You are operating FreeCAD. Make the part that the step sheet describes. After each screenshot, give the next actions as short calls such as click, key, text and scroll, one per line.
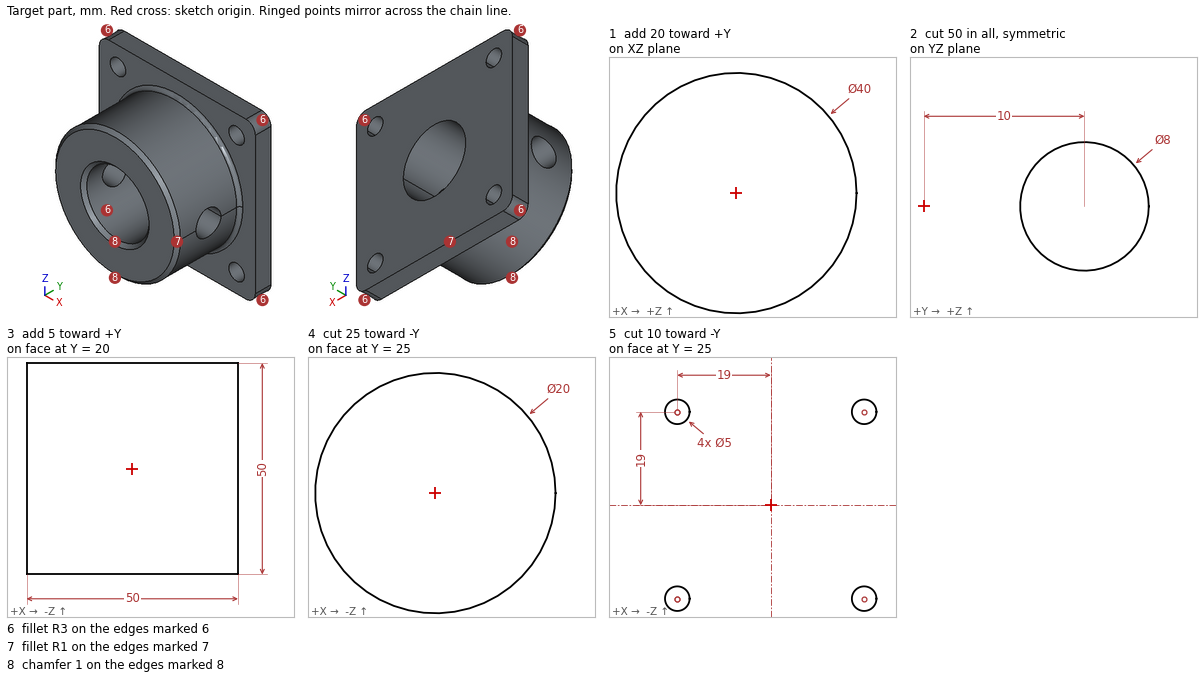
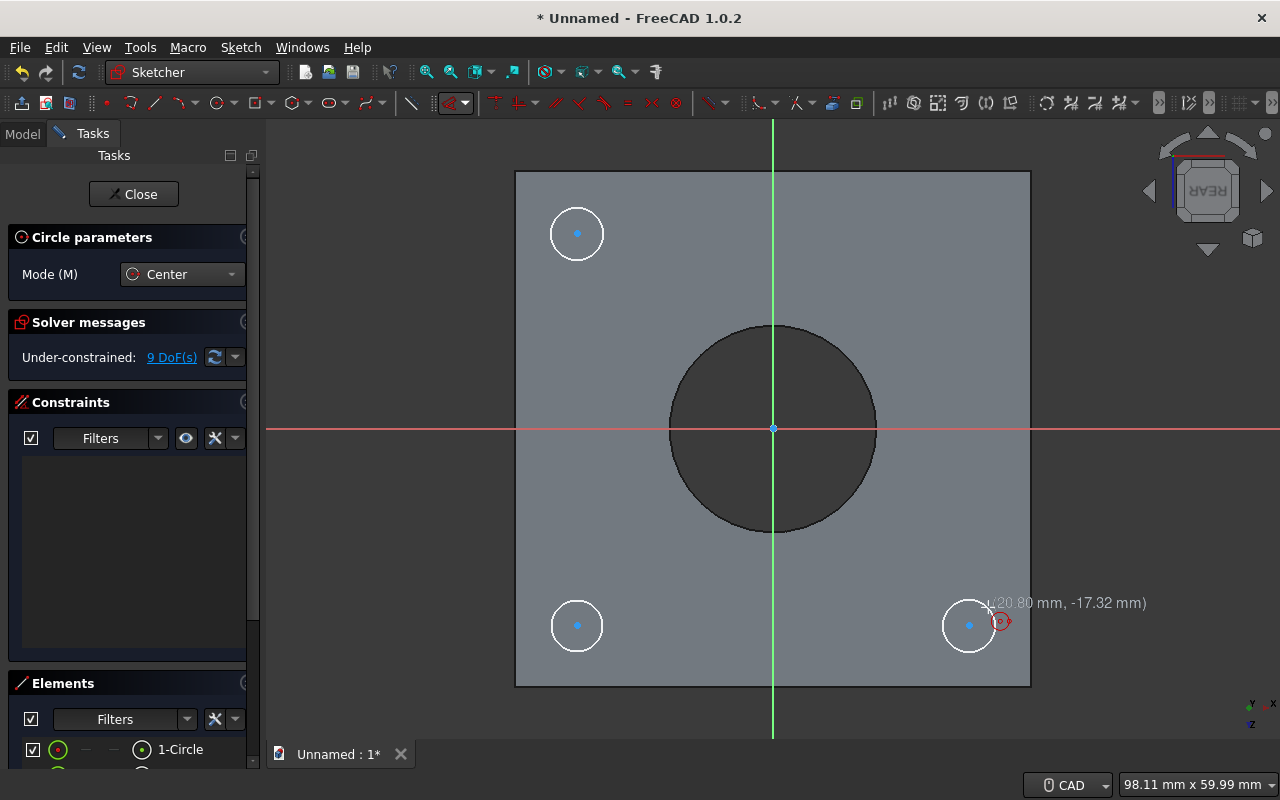
click(969, 233)
click(988, 214)
key(Escape)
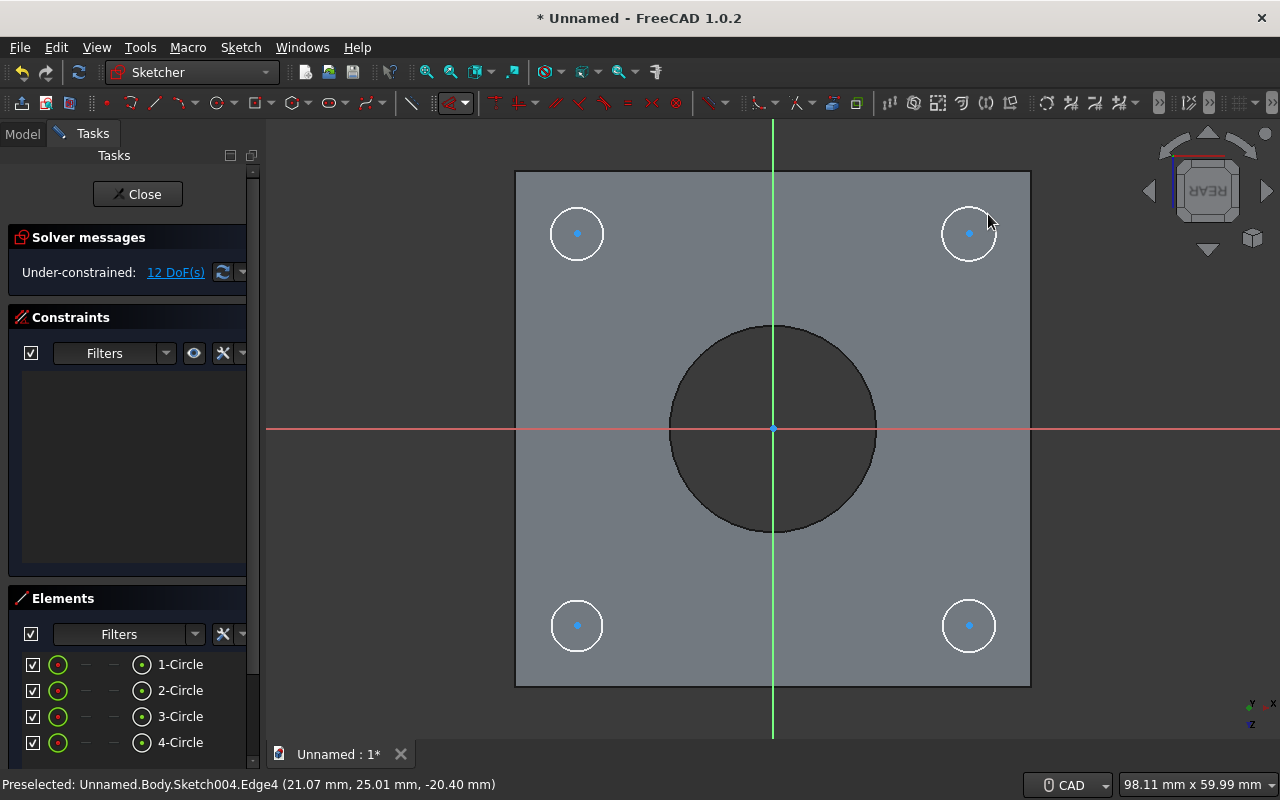
click(595, 215)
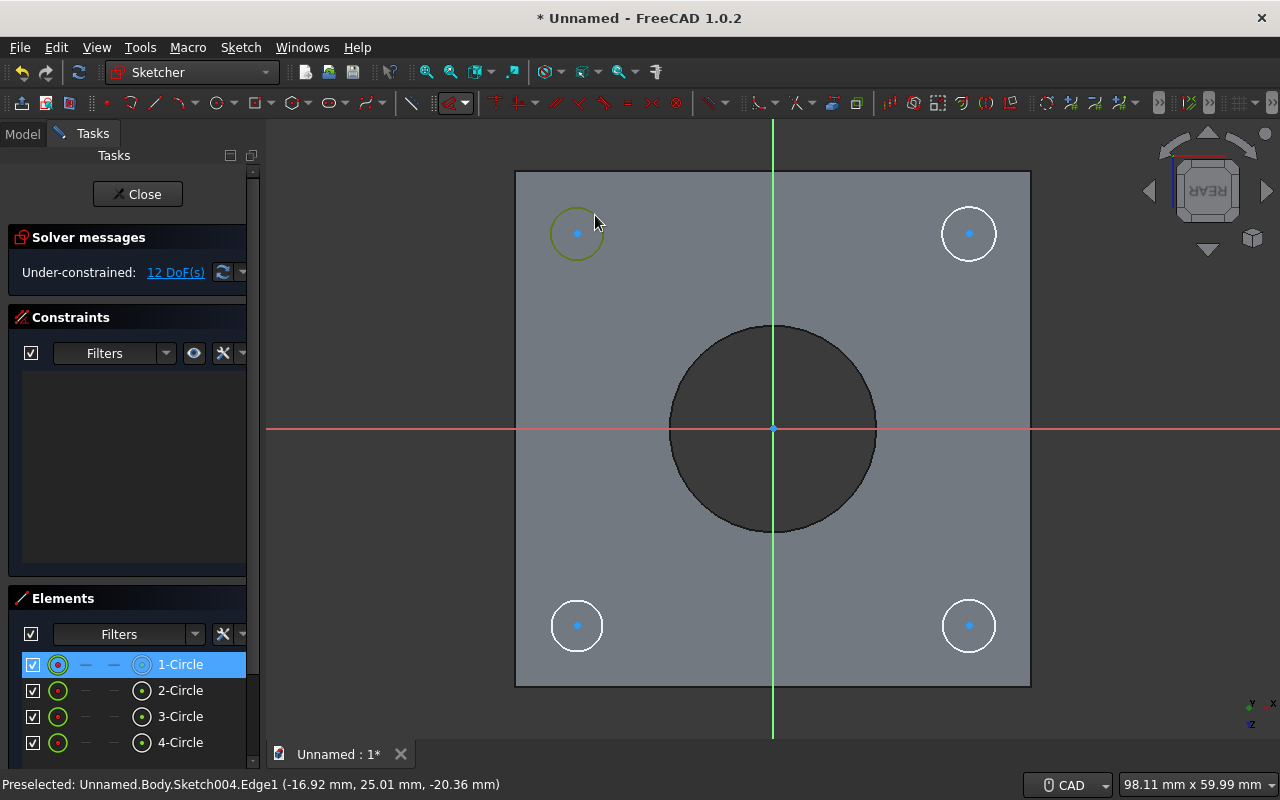
click(595, 608)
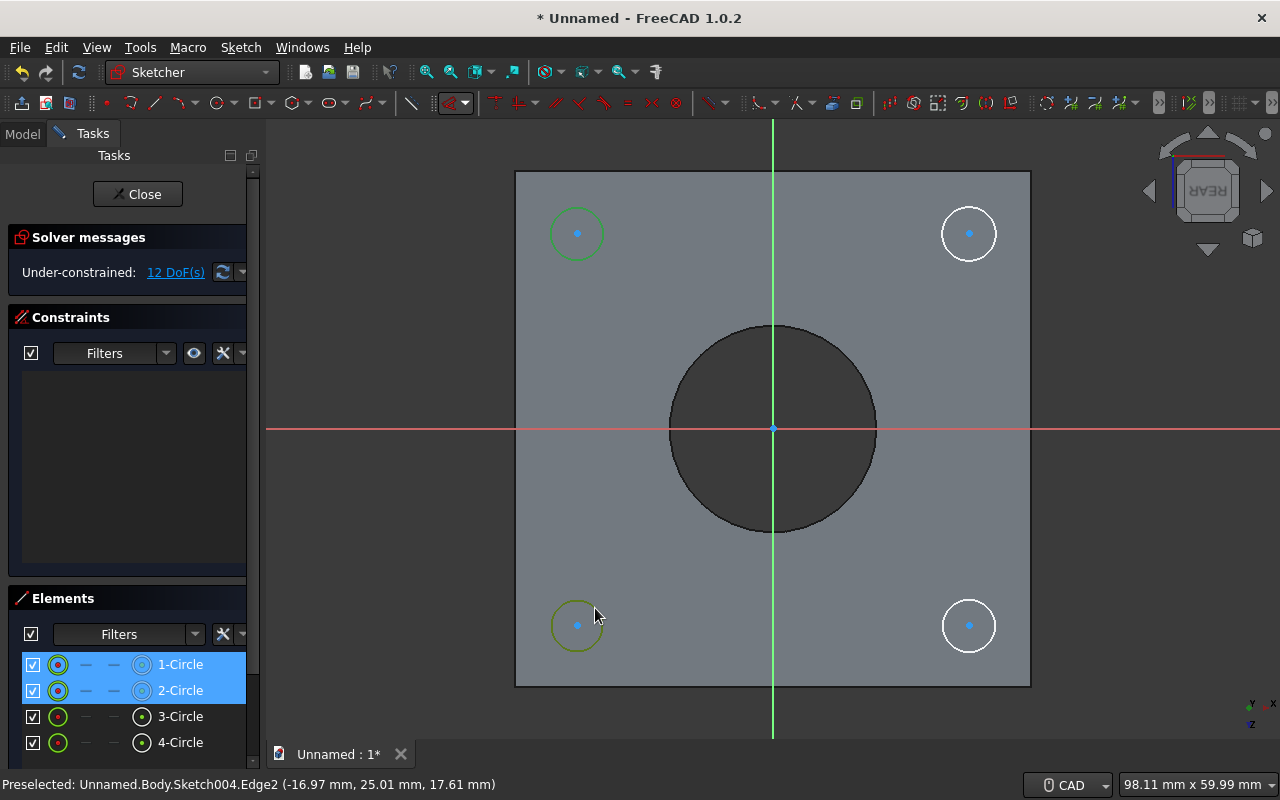
click(987, 607)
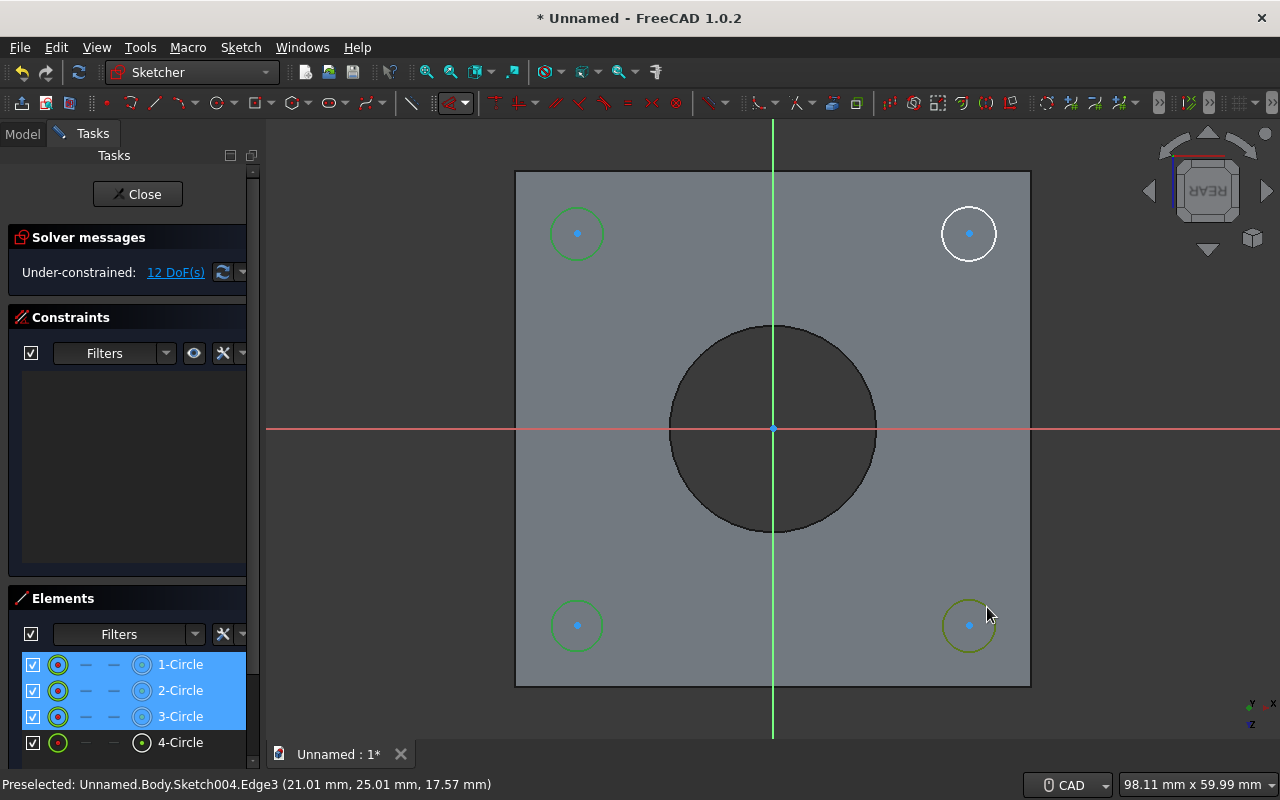
click(988, 215)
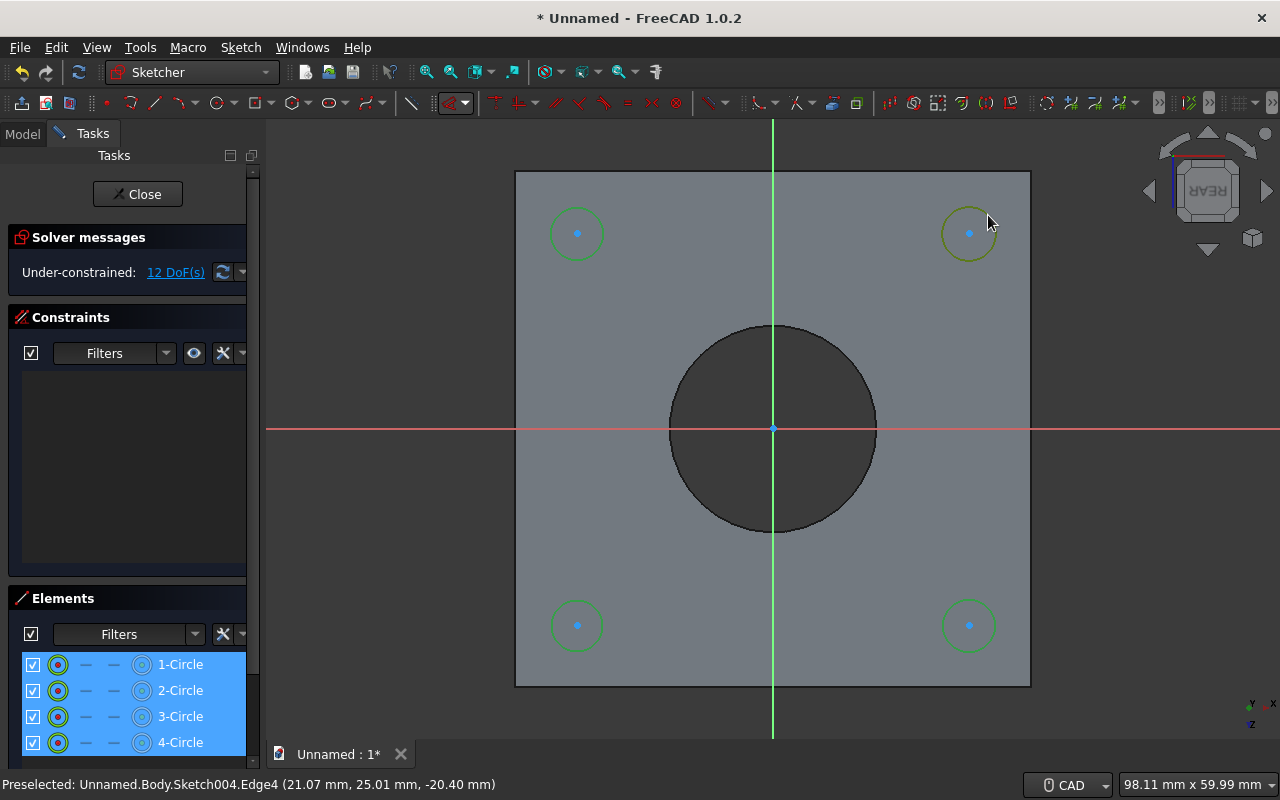
click(628, 104)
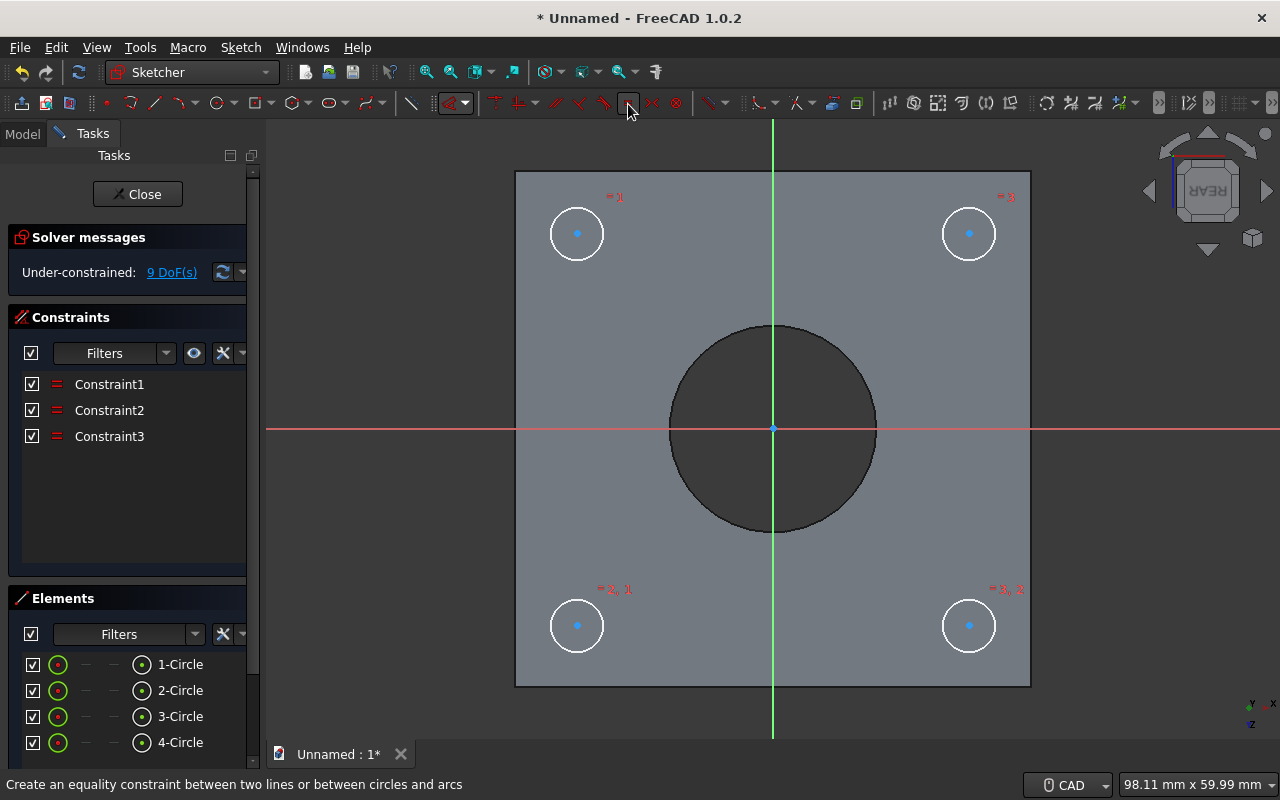
click(577, 234)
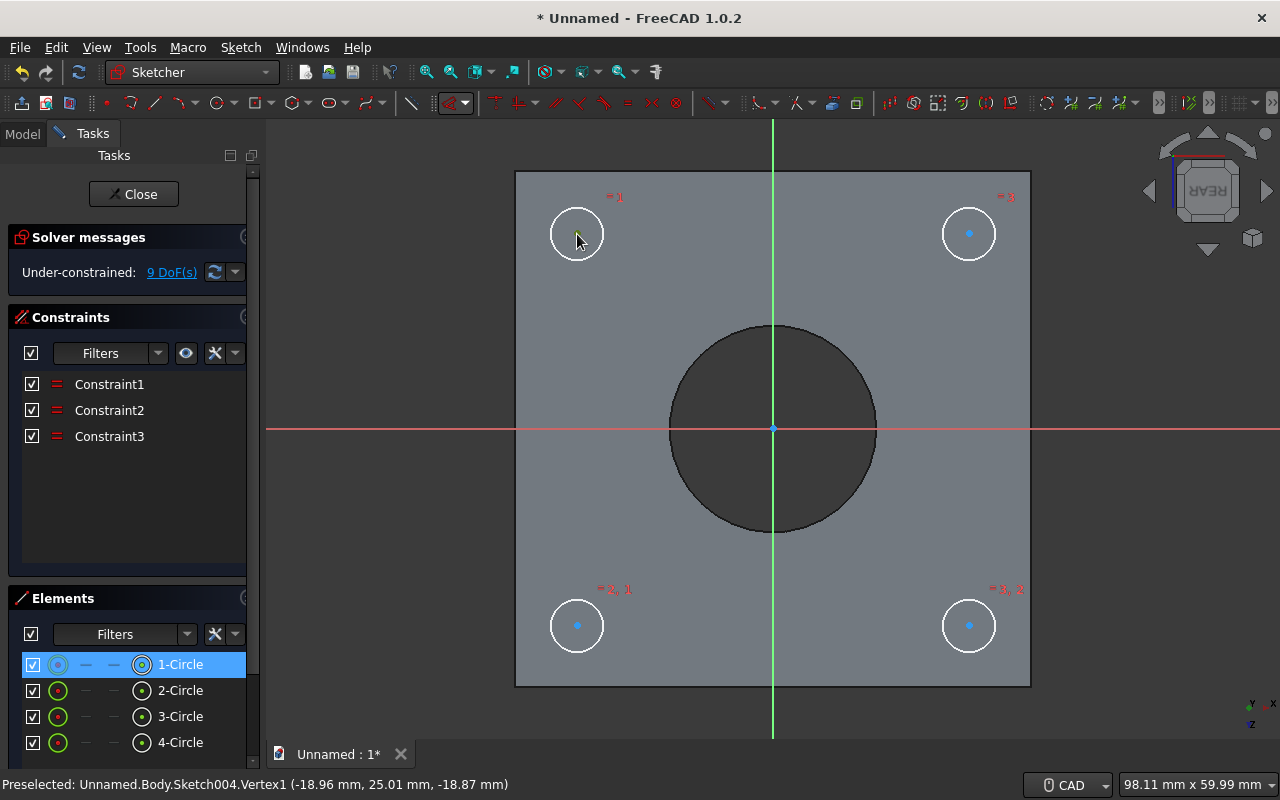
click(577, 626)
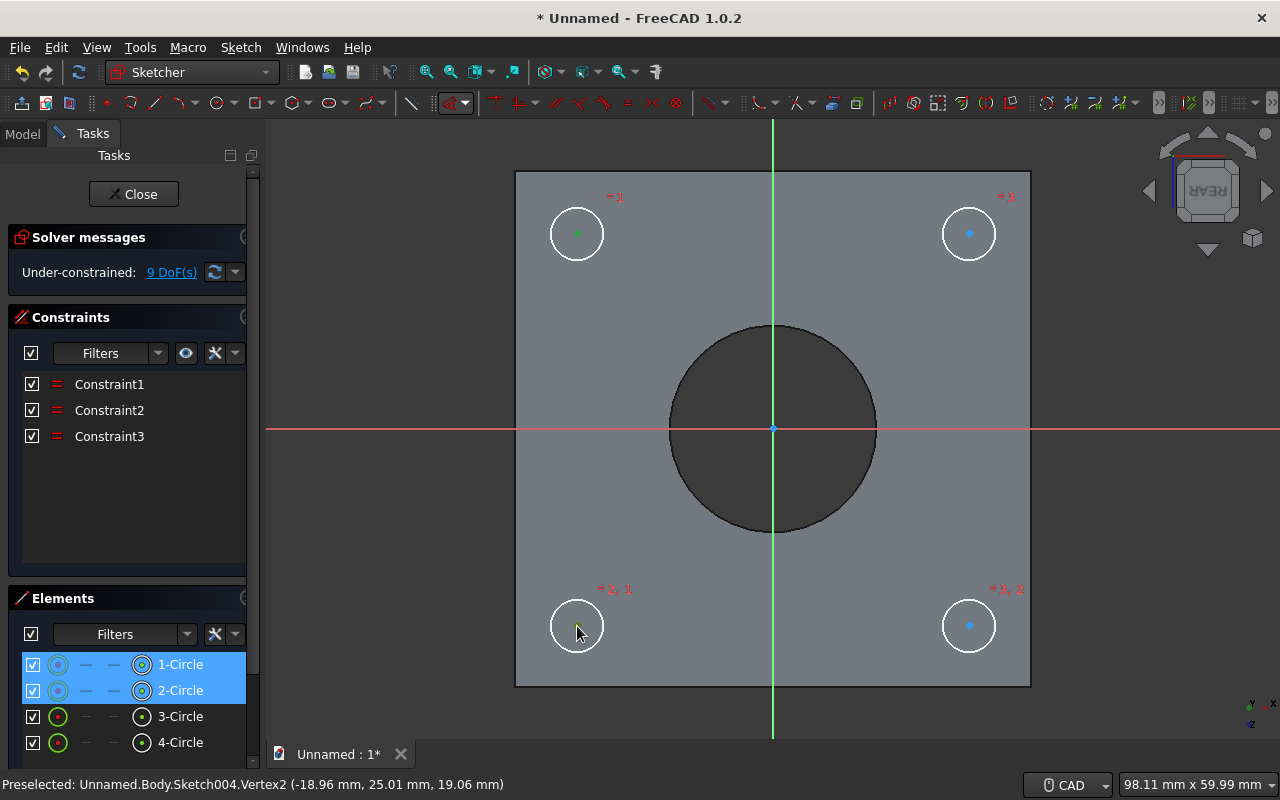
click(353, 429)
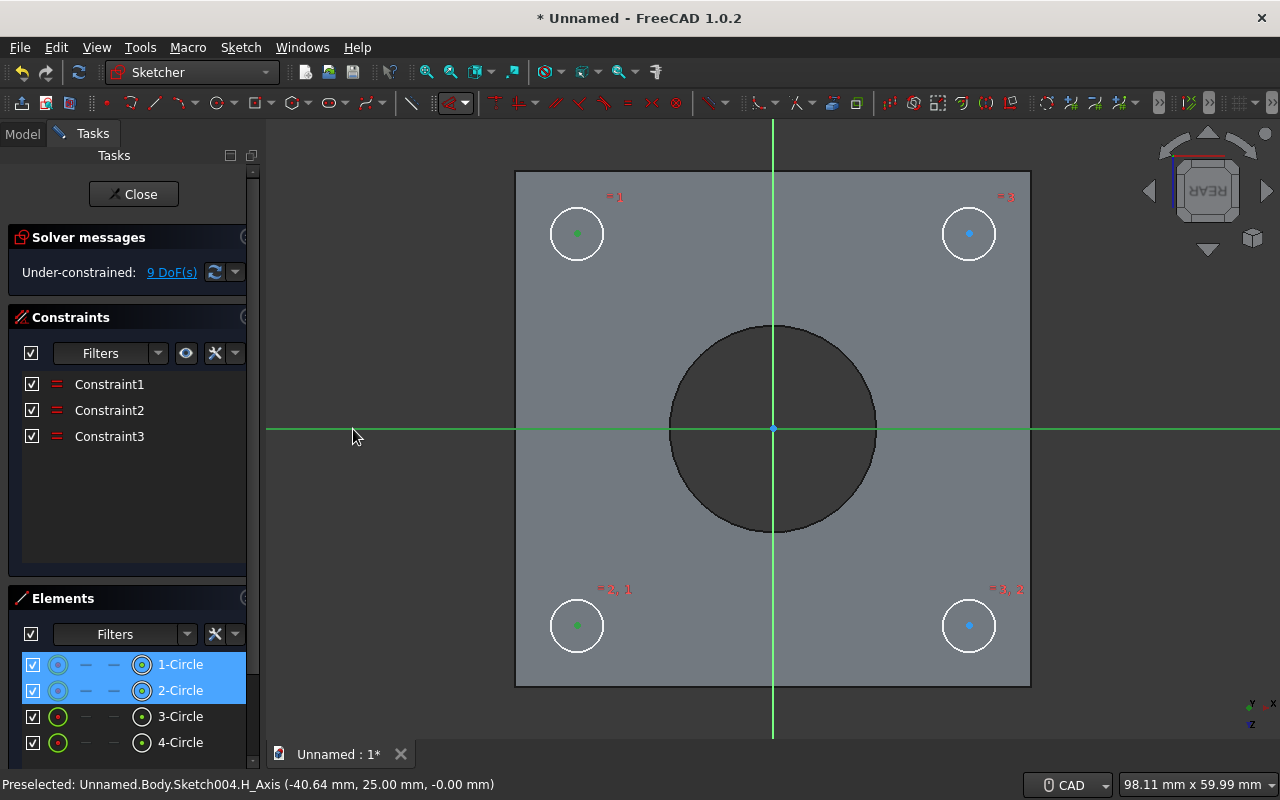
click(652, 104)